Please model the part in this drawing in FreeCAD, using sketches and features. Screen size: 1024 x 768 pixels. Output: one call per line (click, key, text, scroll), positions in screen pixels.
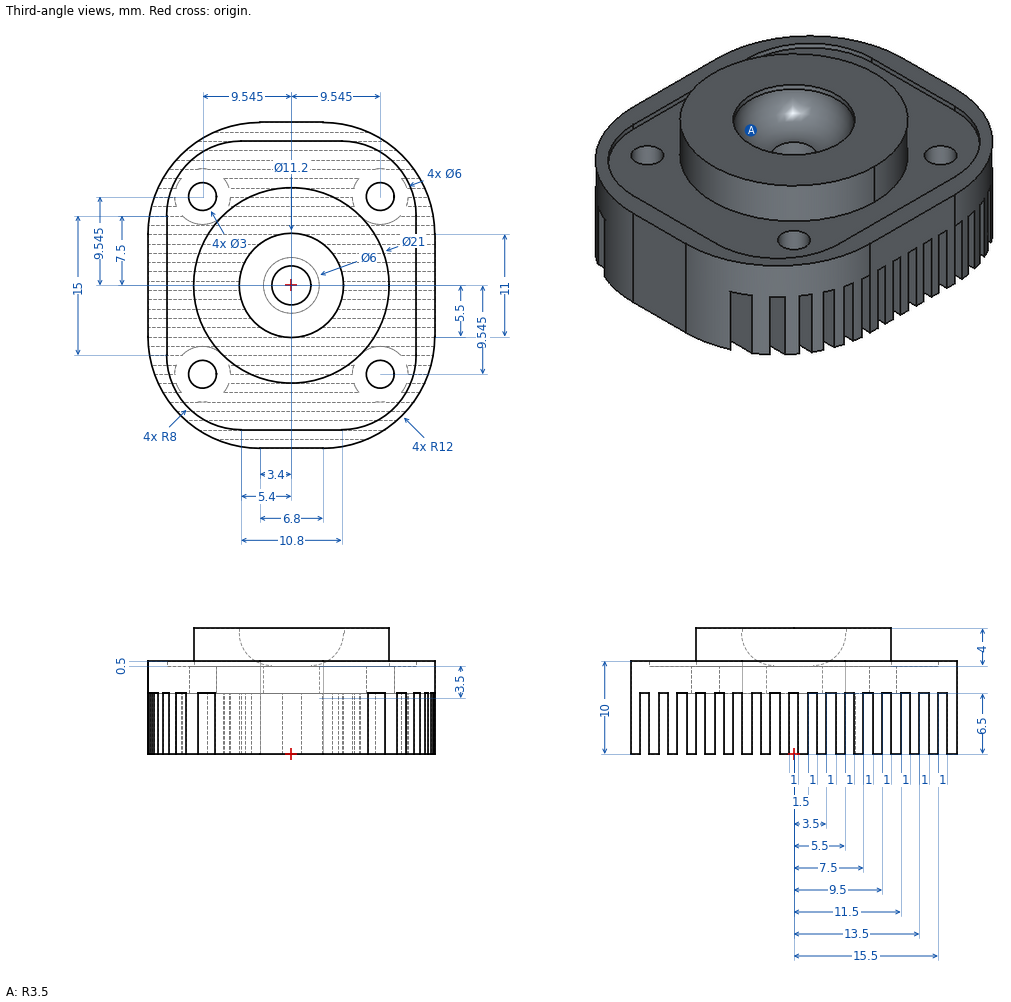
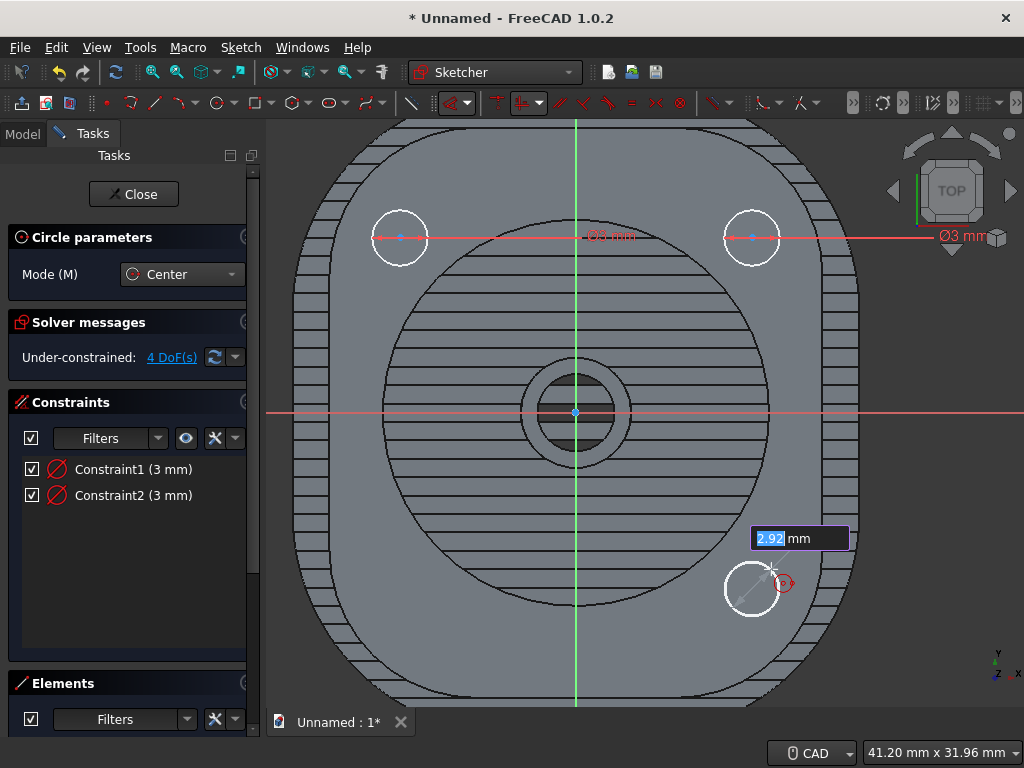
text(3)
key(Return)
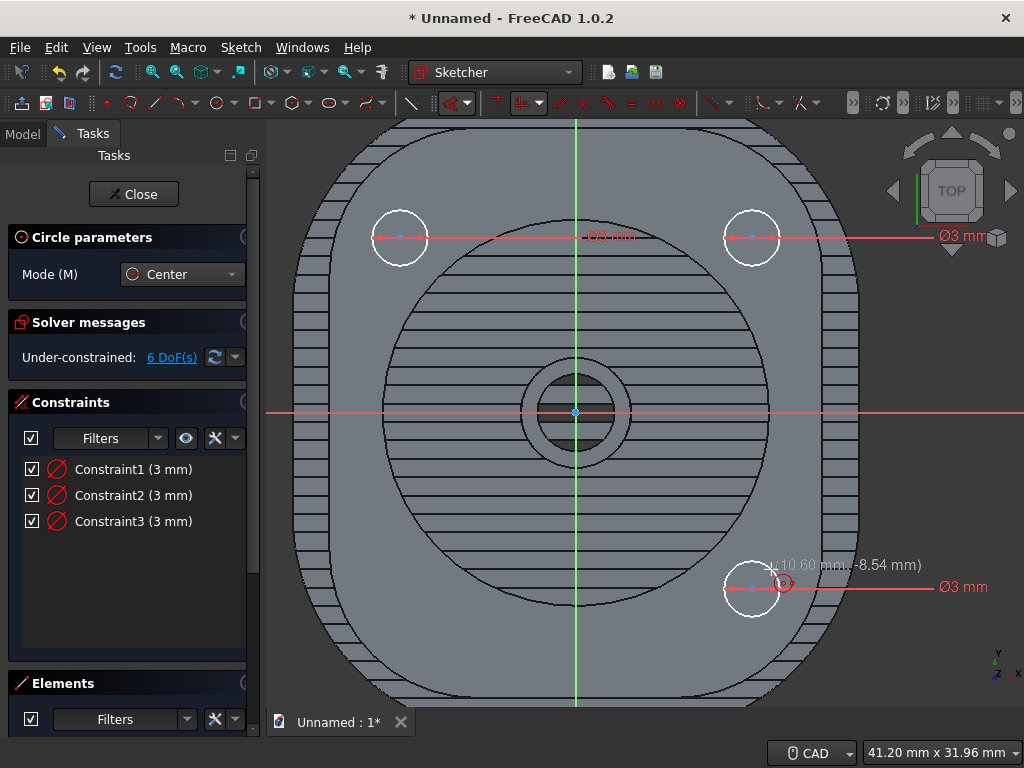
click(400, 588)
move(420, 569)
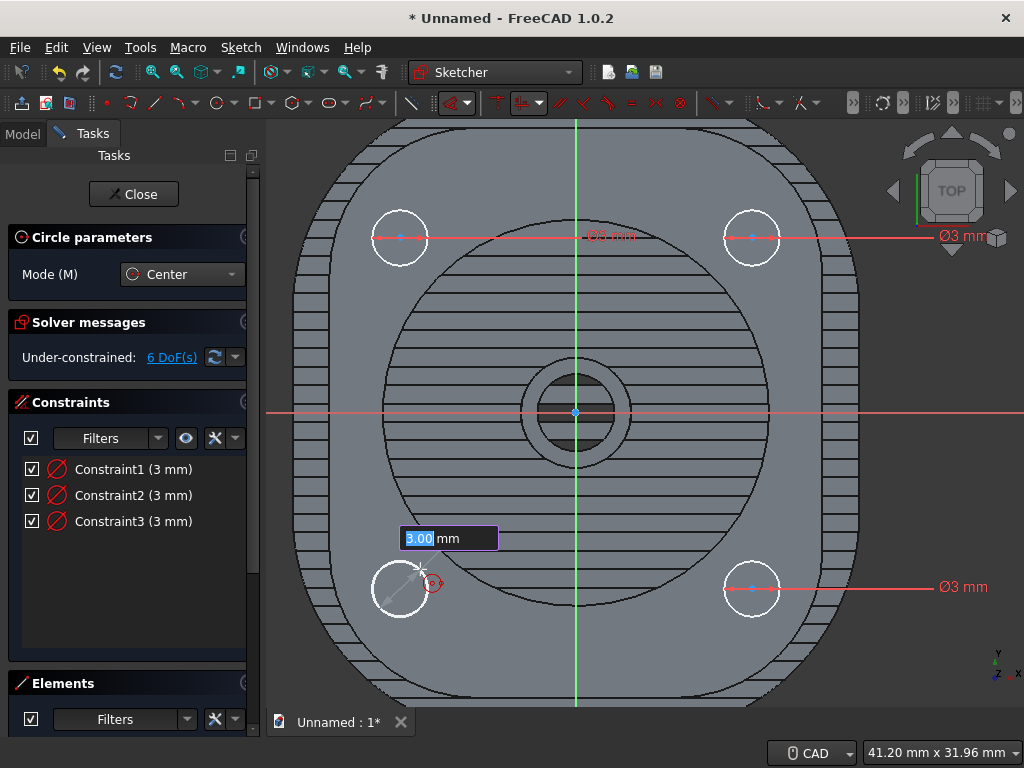
text(3)
key(Return)
key(Escape)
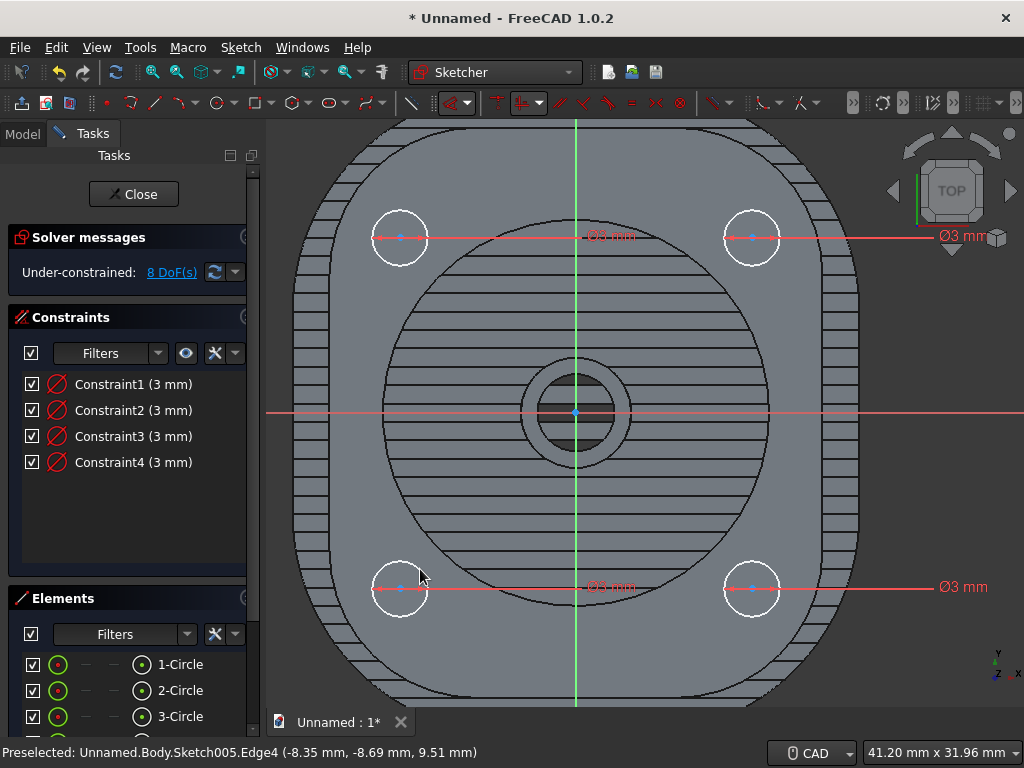
click(400, 238)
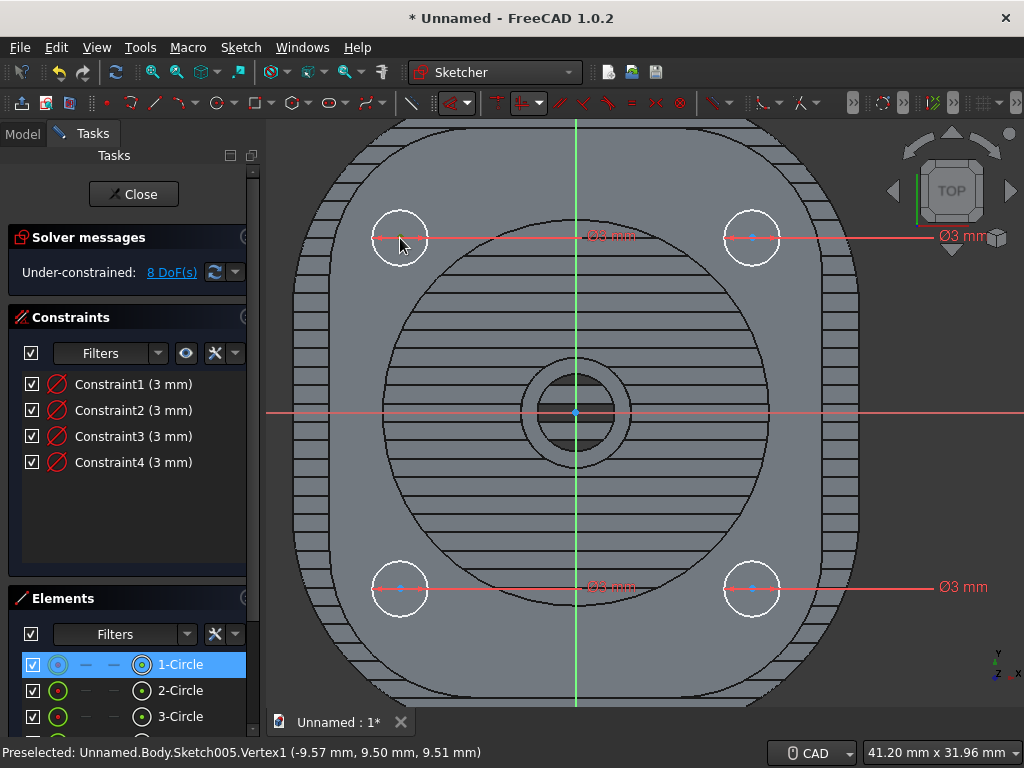
click(752, 238)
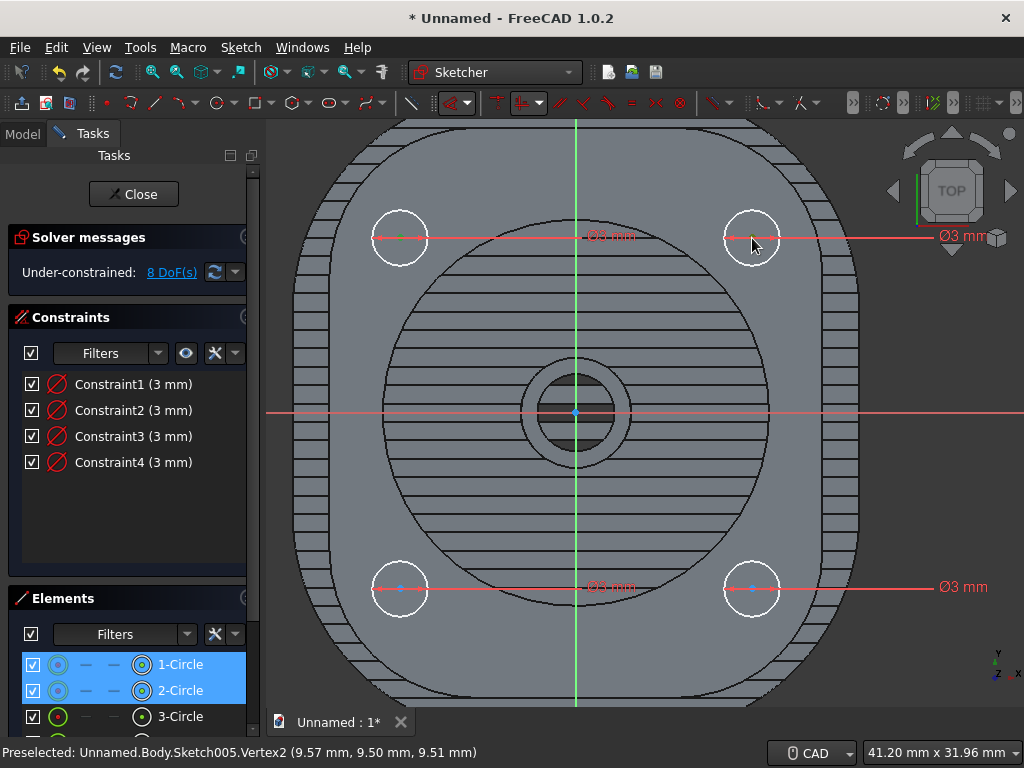
key(h)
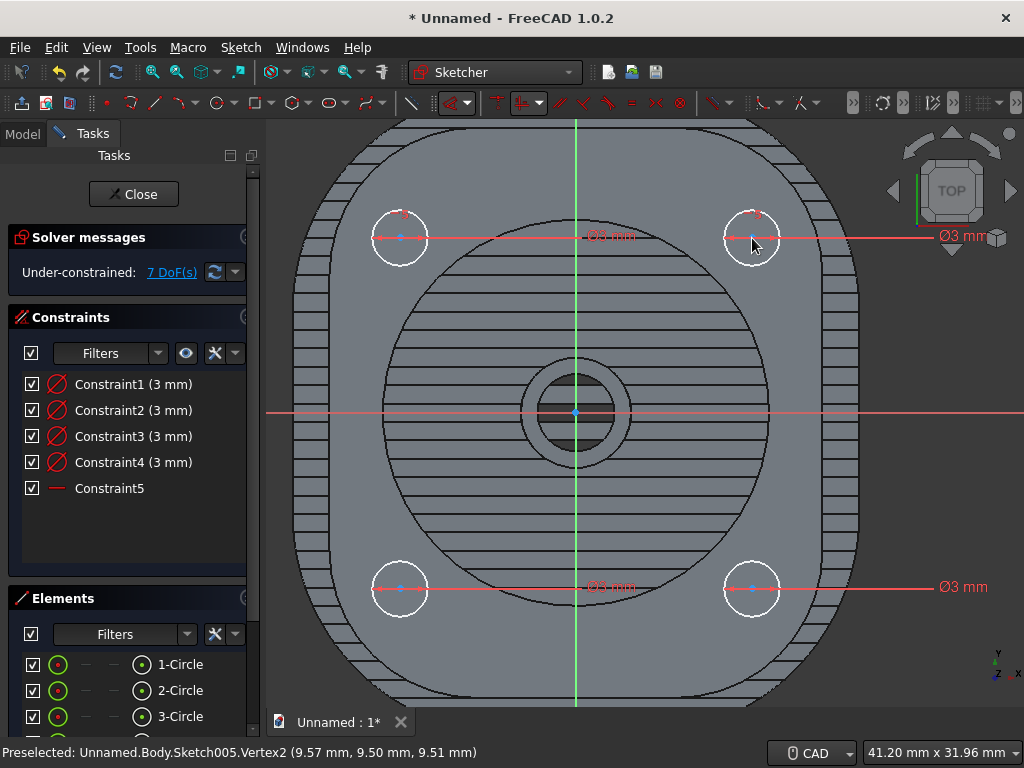
click(752, 238)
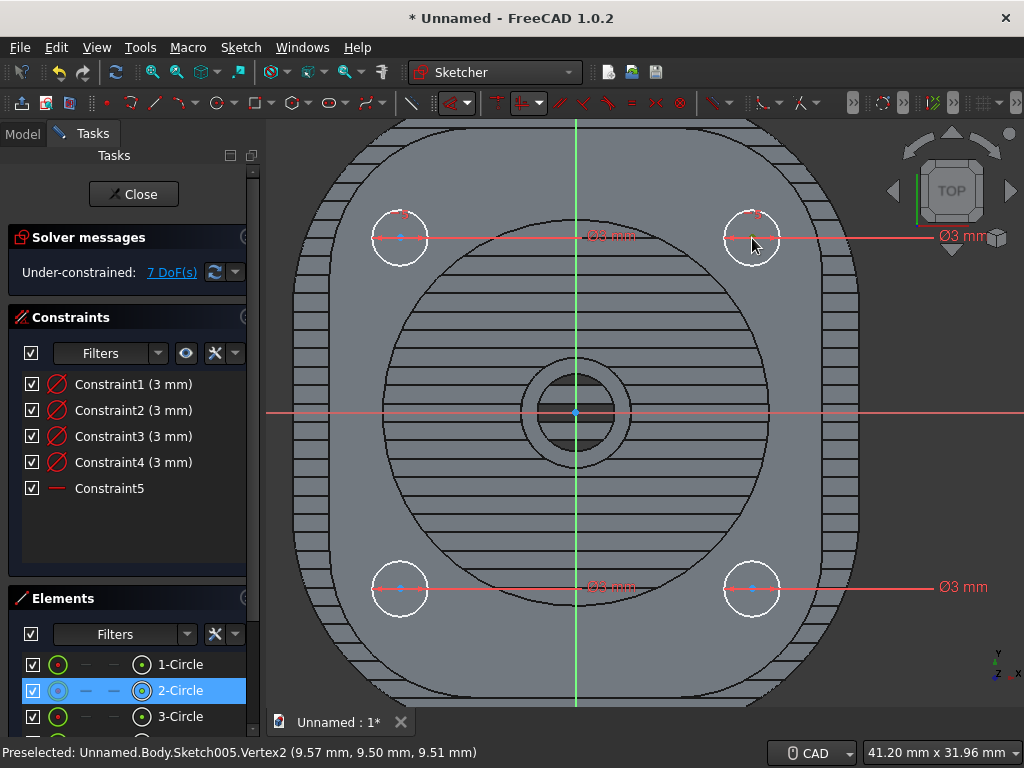
click(752, 589)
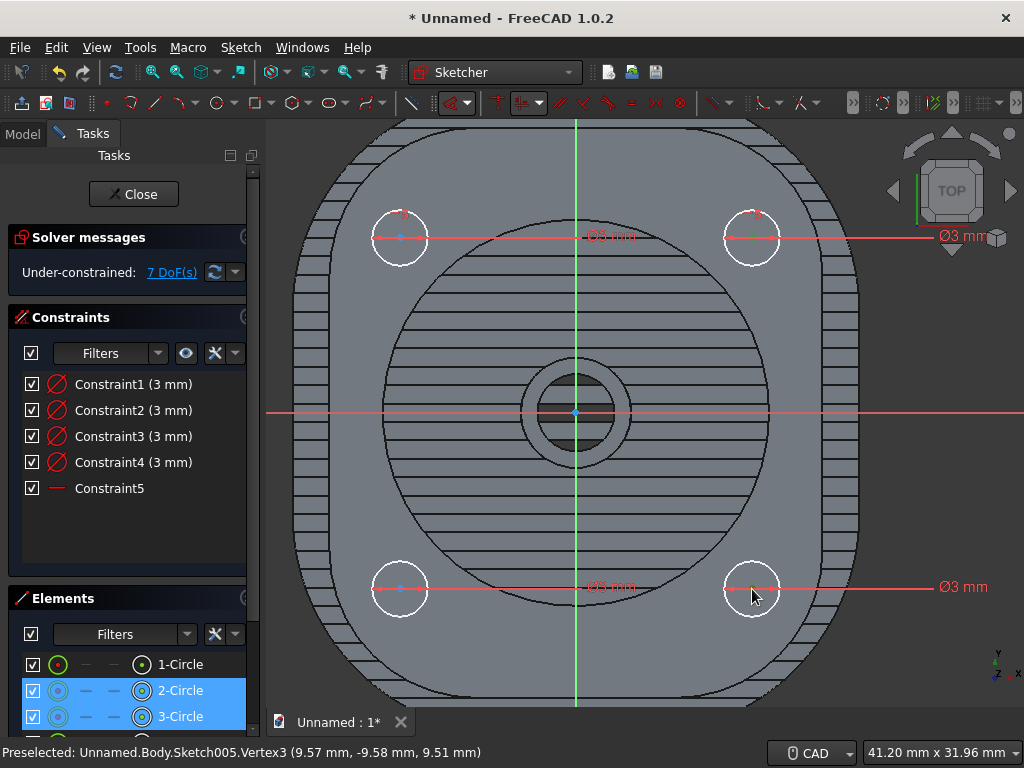
key(v)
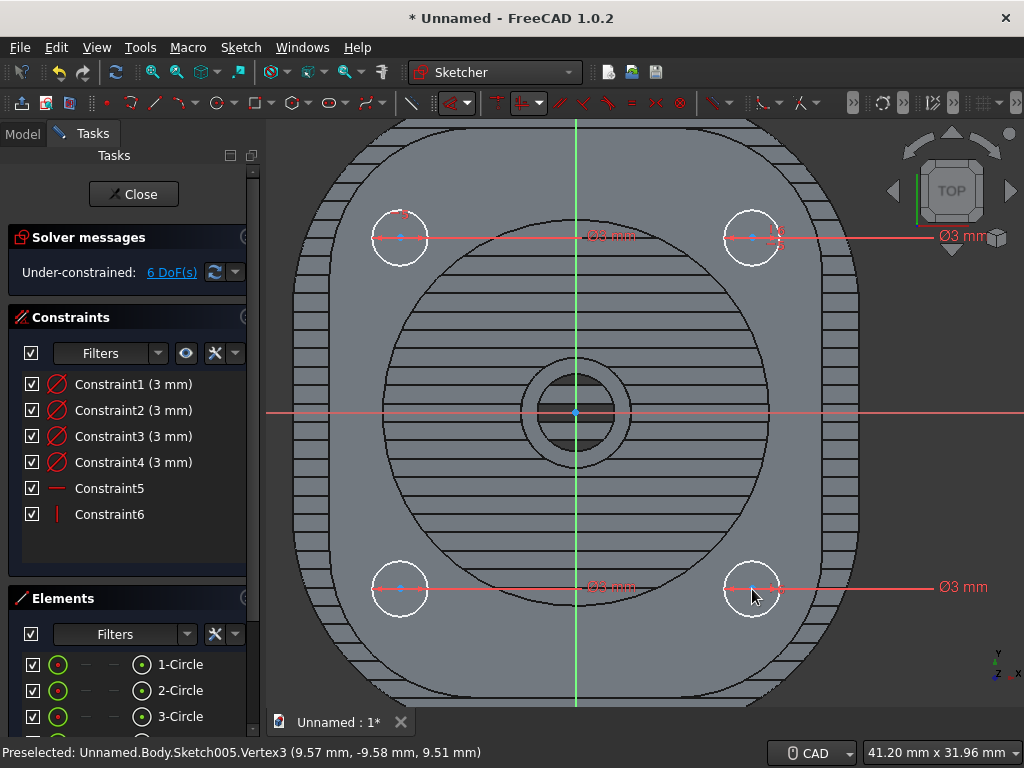
click(400, 238)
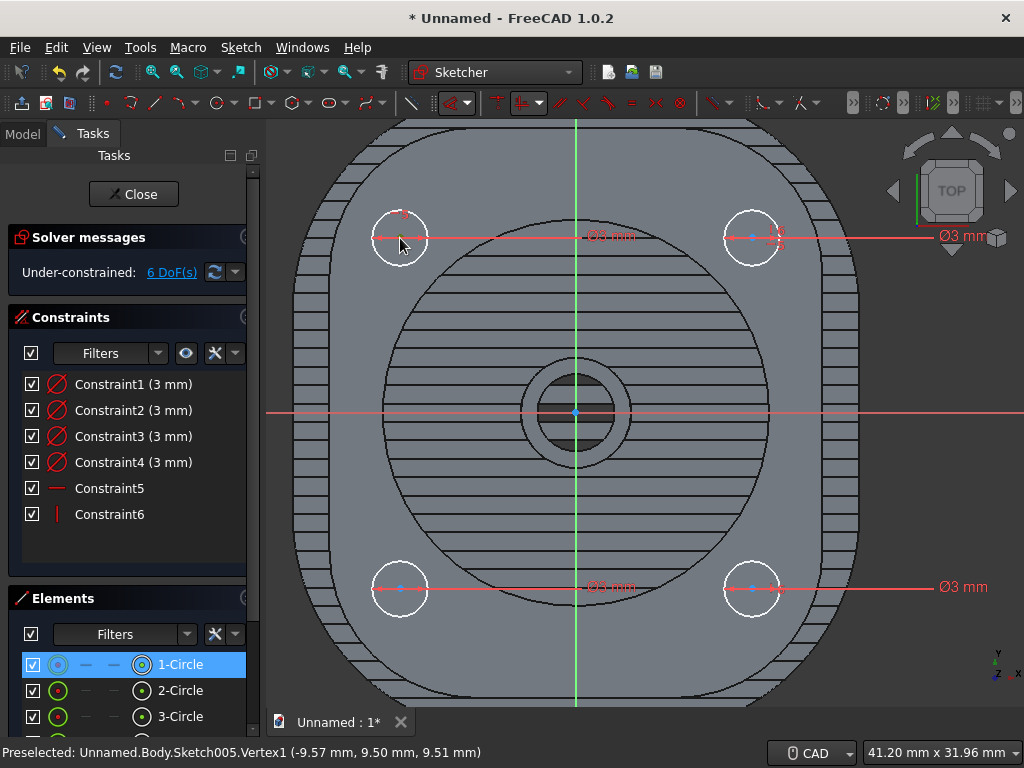
click(400, 589)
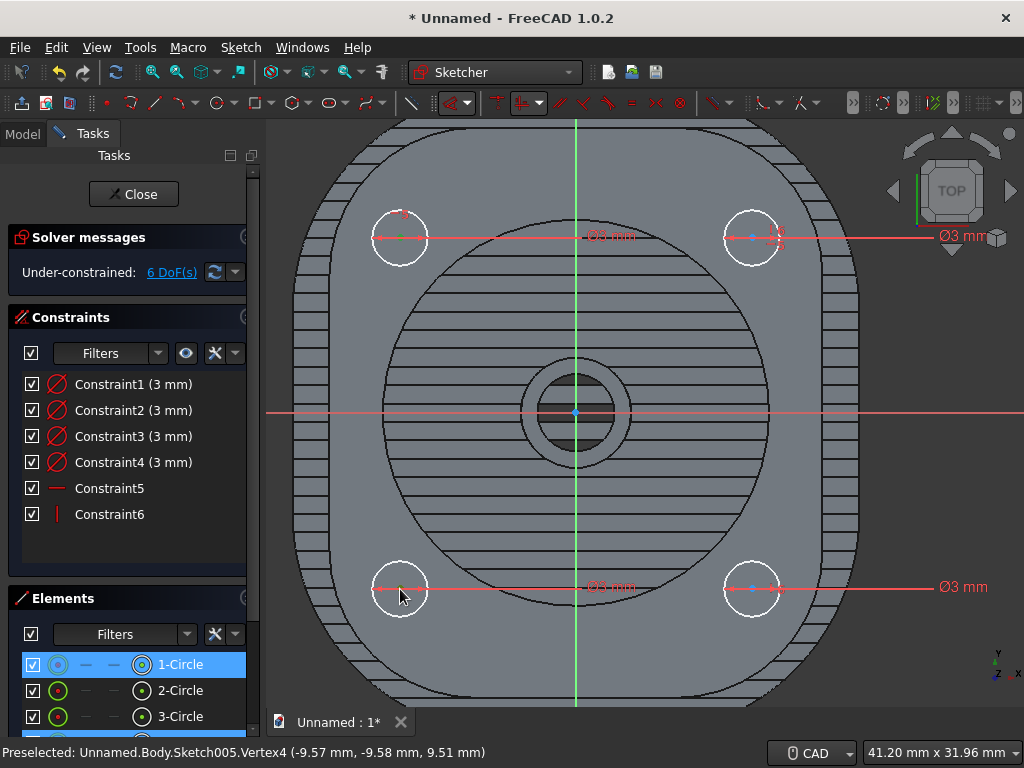
click(542, 104)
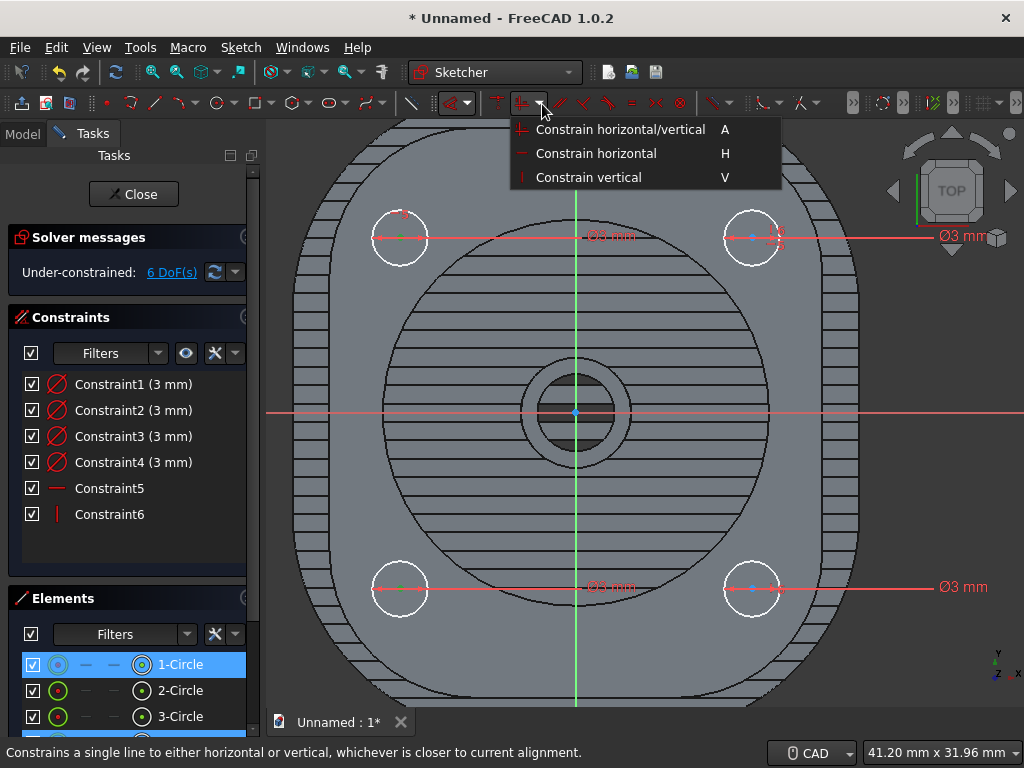
click(646, 177)